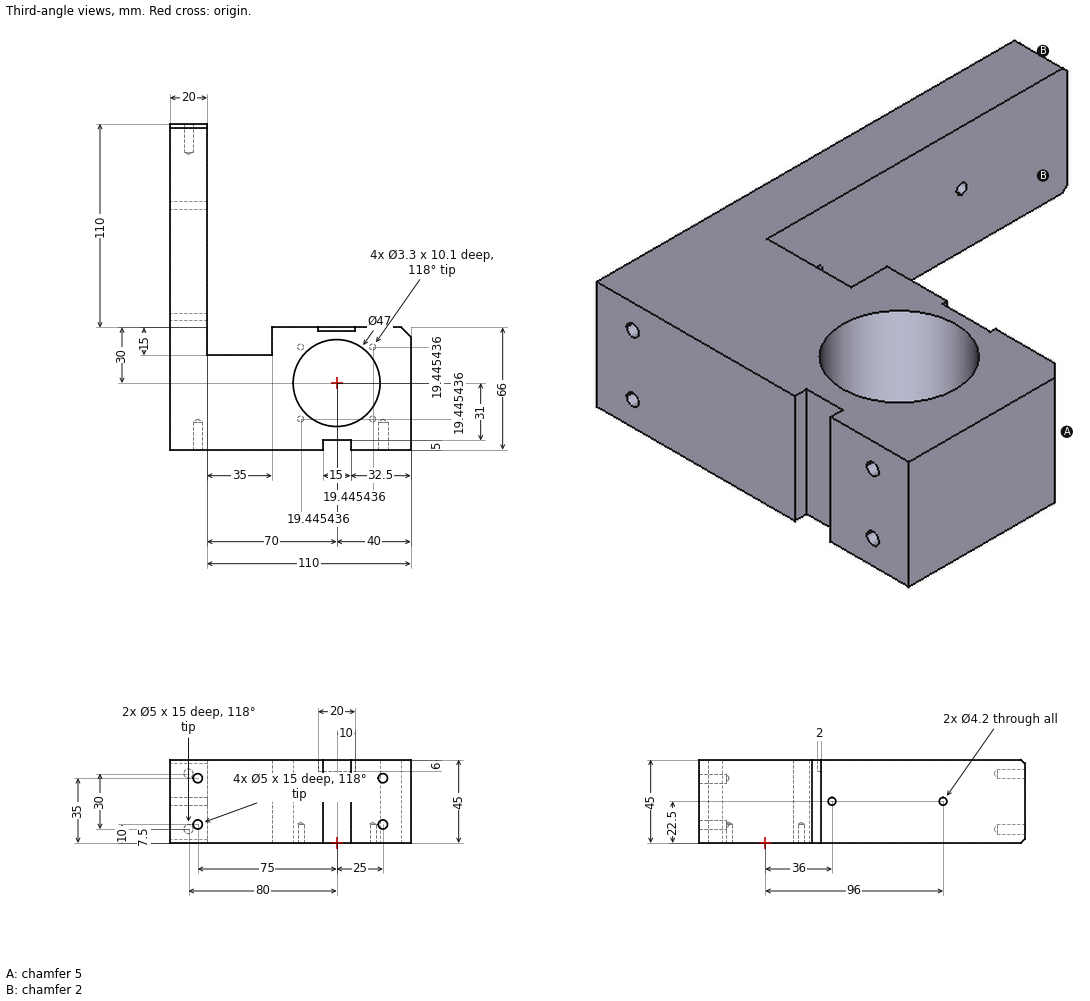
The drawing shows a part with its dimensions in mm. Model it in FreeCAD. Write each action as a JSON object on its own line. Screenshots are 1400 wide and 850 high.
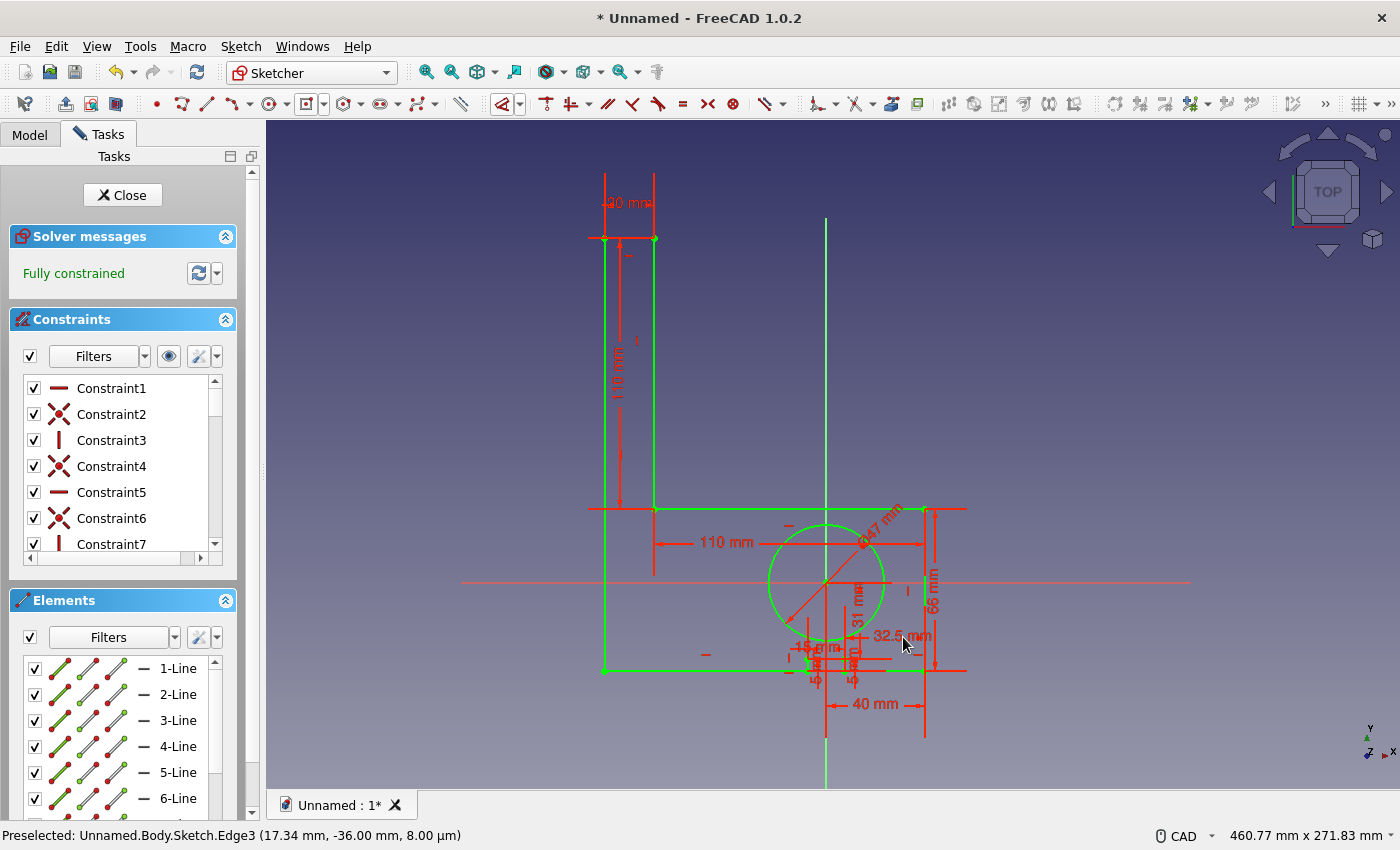
{"action": "left_click", "coordinate": [123, 195]}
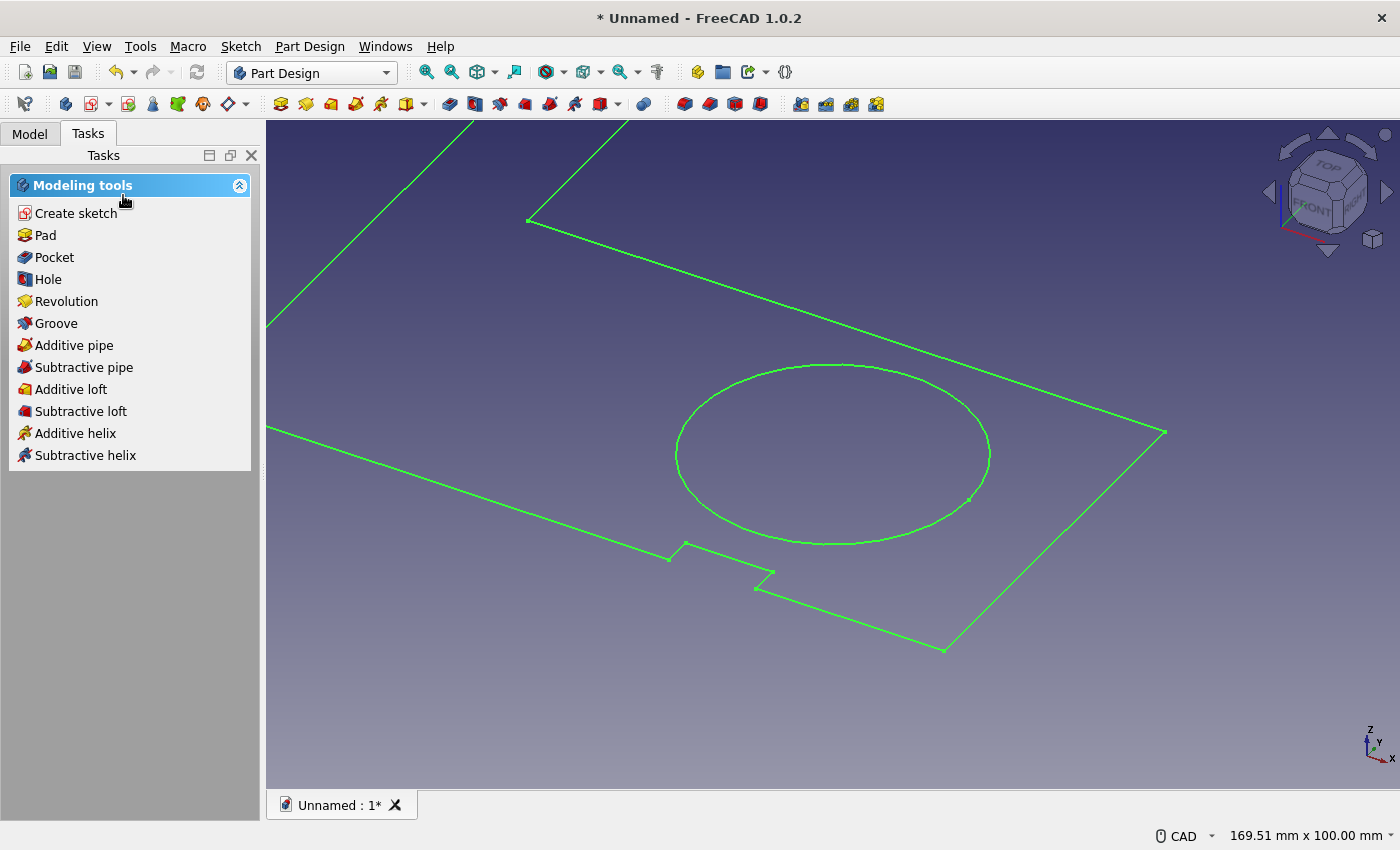
{"action": "left_click", "coordinate": [281, 104]}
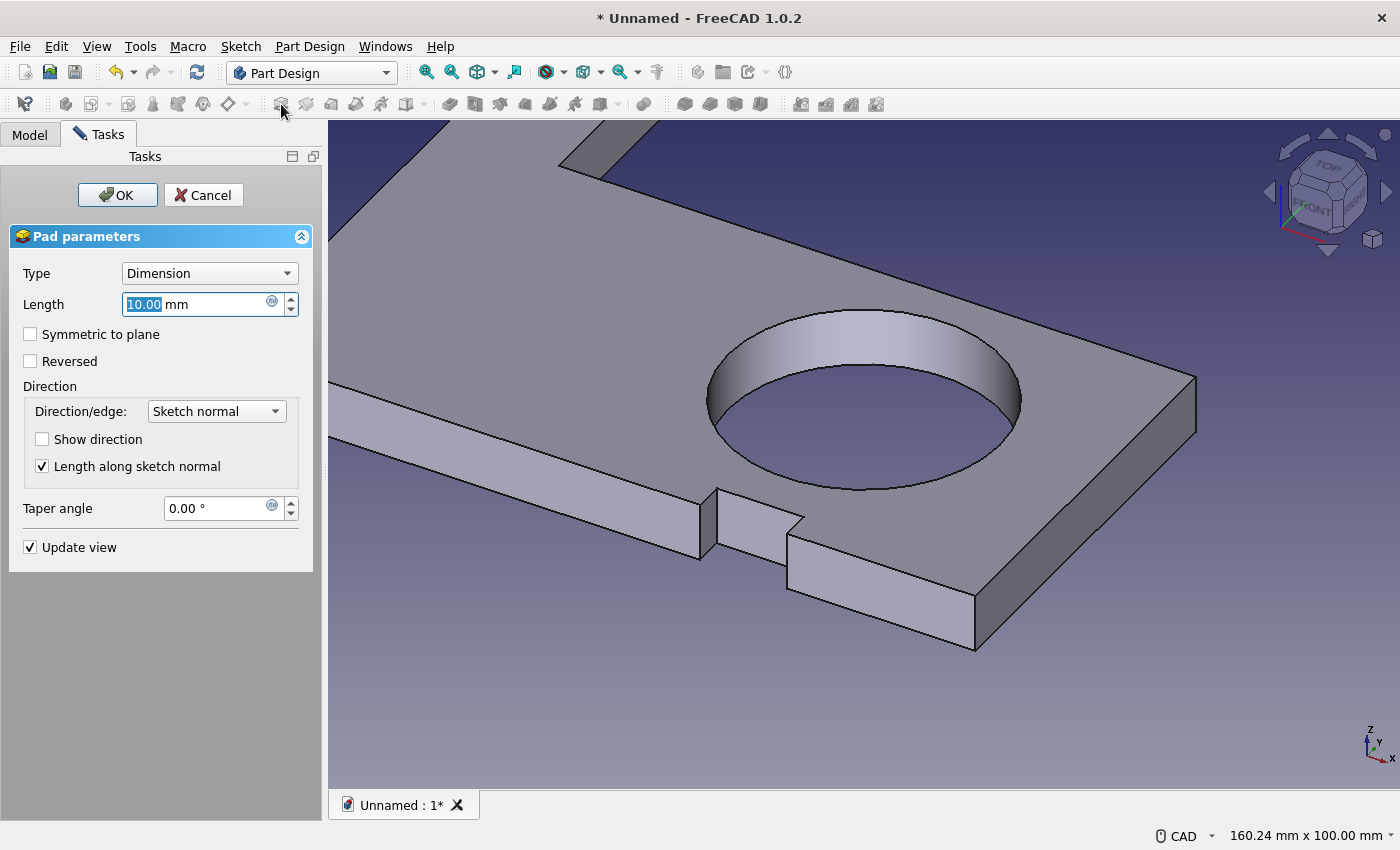
{"action": "type", "text": "45"}
{"action": "key", "text": "Tab"}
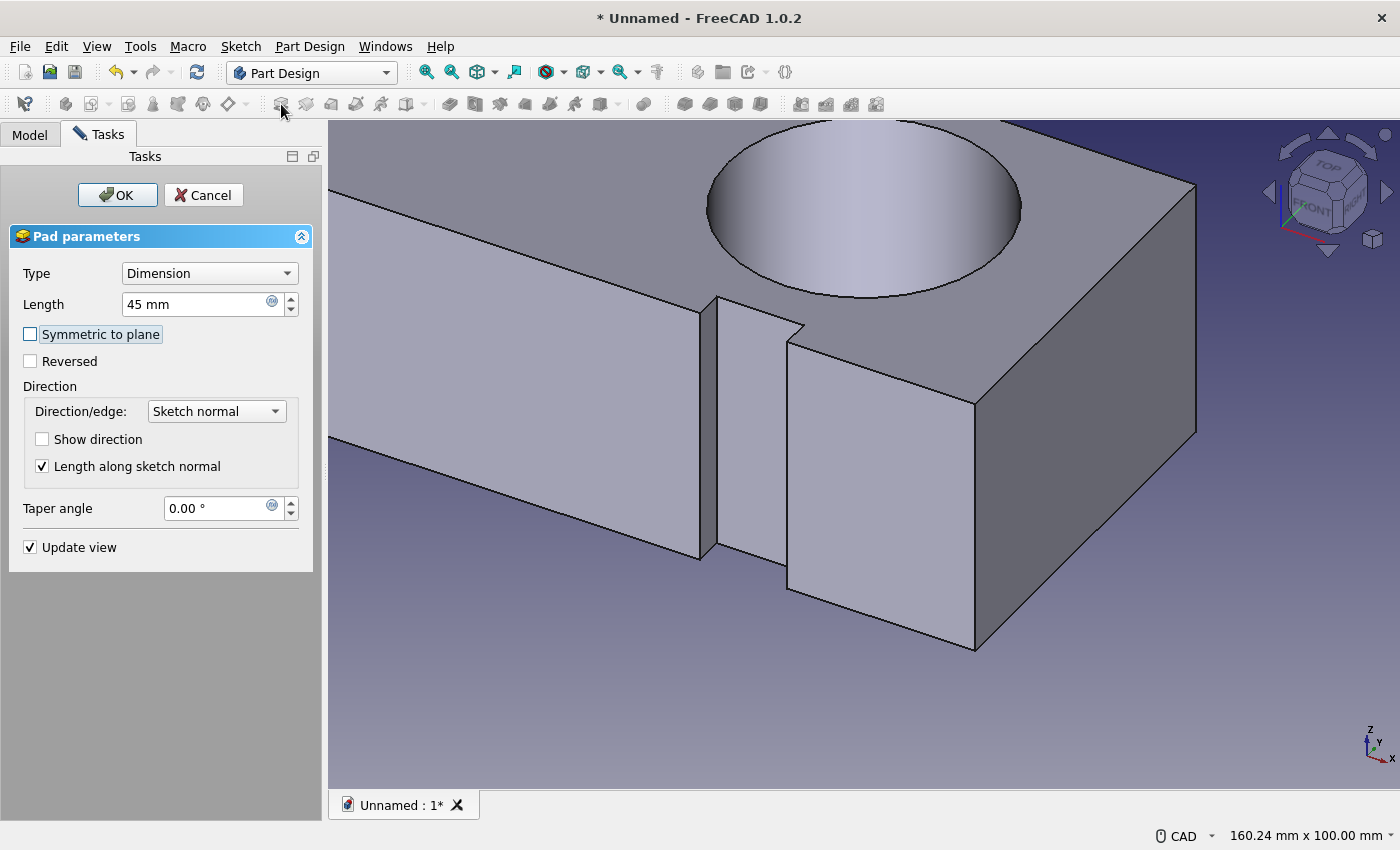
{"action": "left_click", "coordinate": [118, 195]}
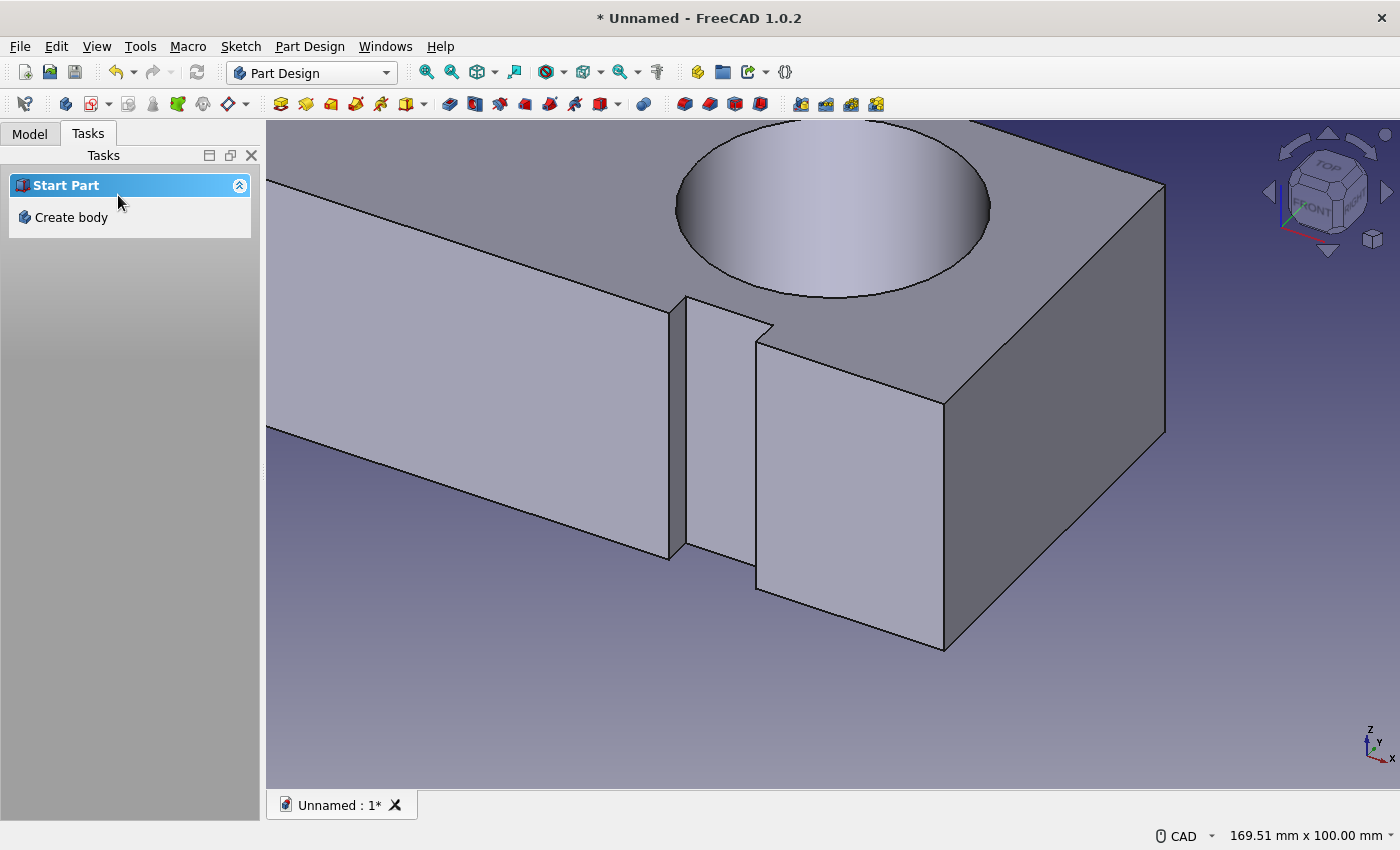
{"action": "key", "text": "v f"}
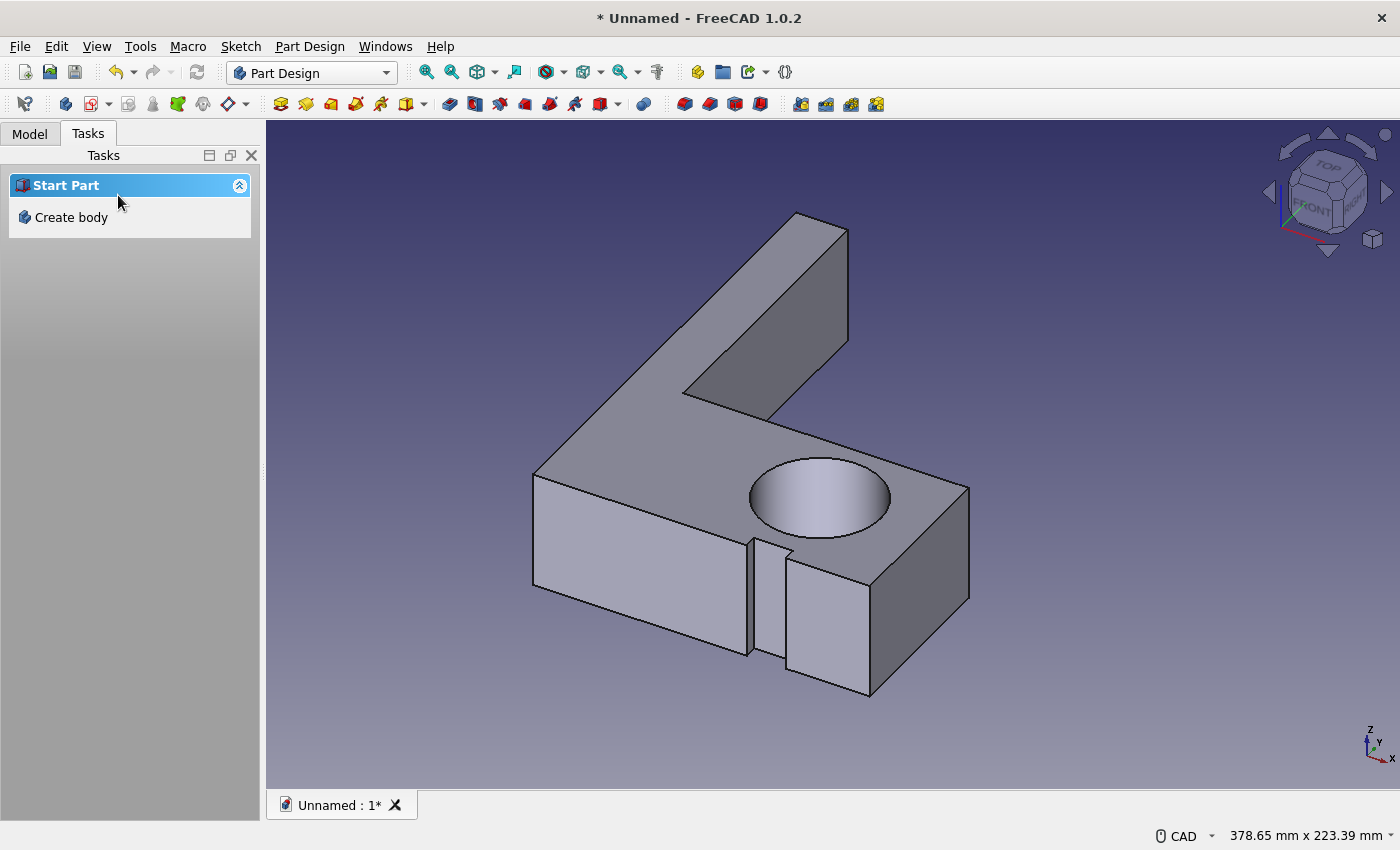
{"action": "left_click", "coordinate": [670, 574]}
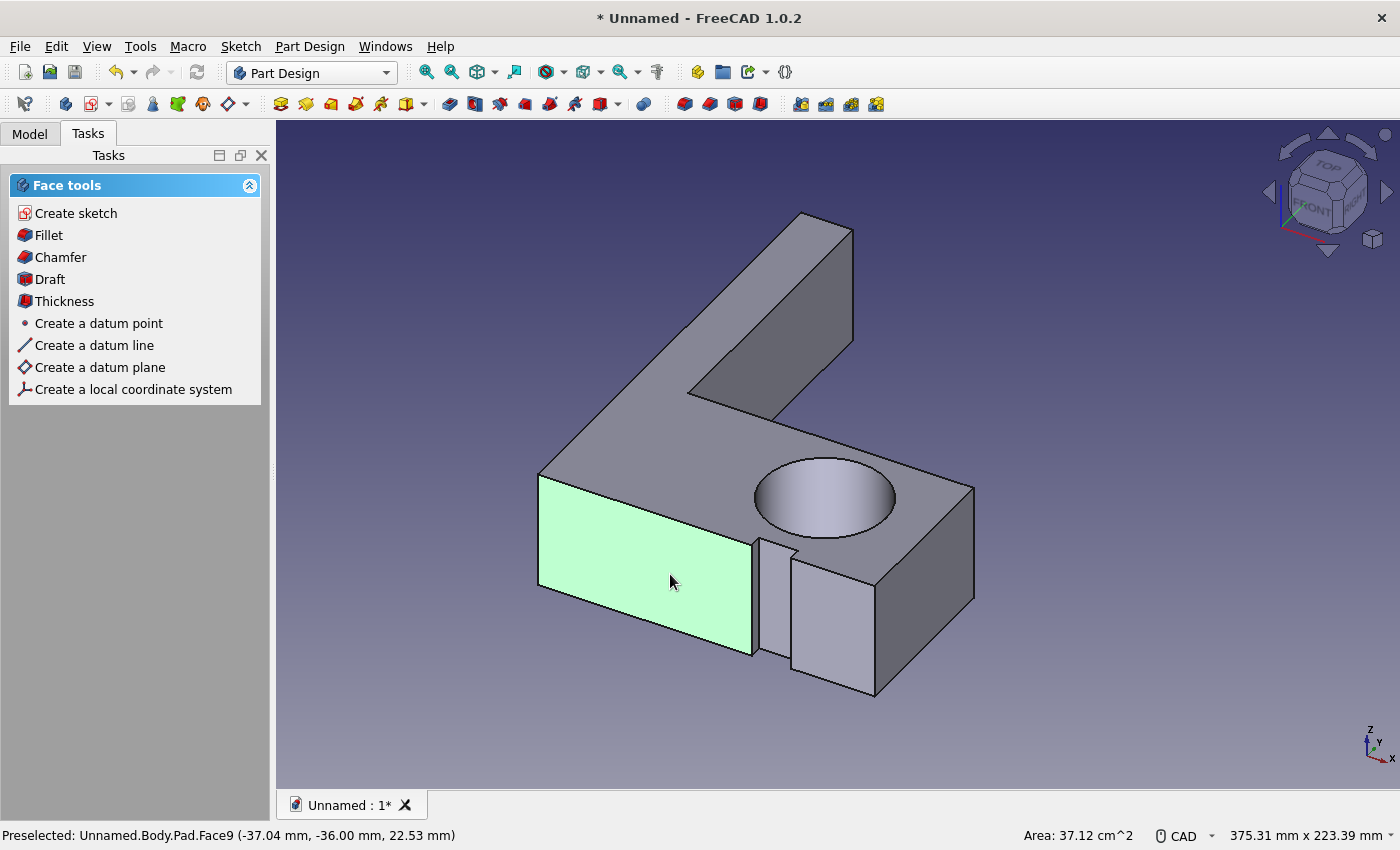
{"action": "left_click", "coordinate": [90, 104]}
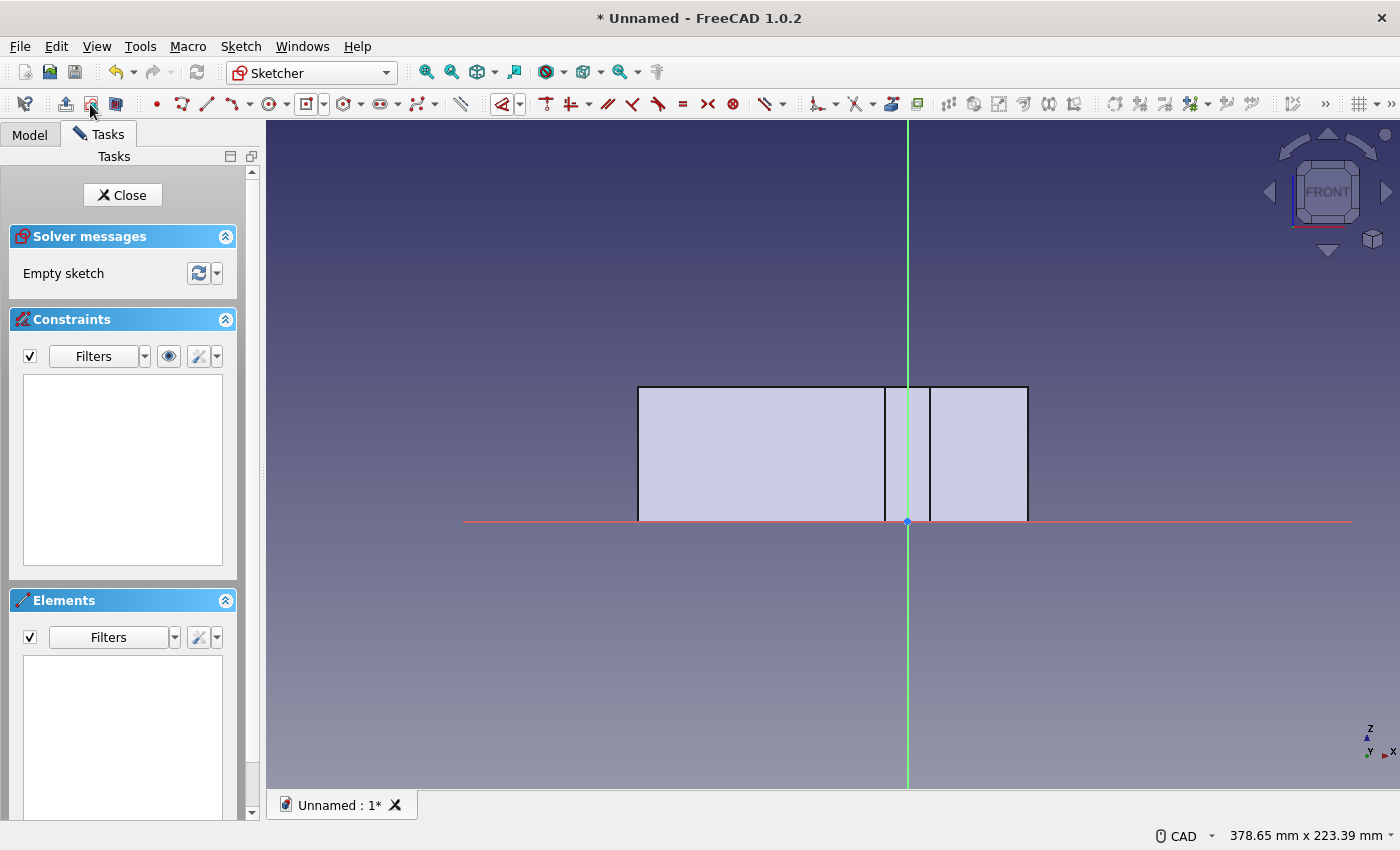
{"action": "scroll", "coordinate": [889, 475], "scroll_direction": "up", "scroll_amount": 4}